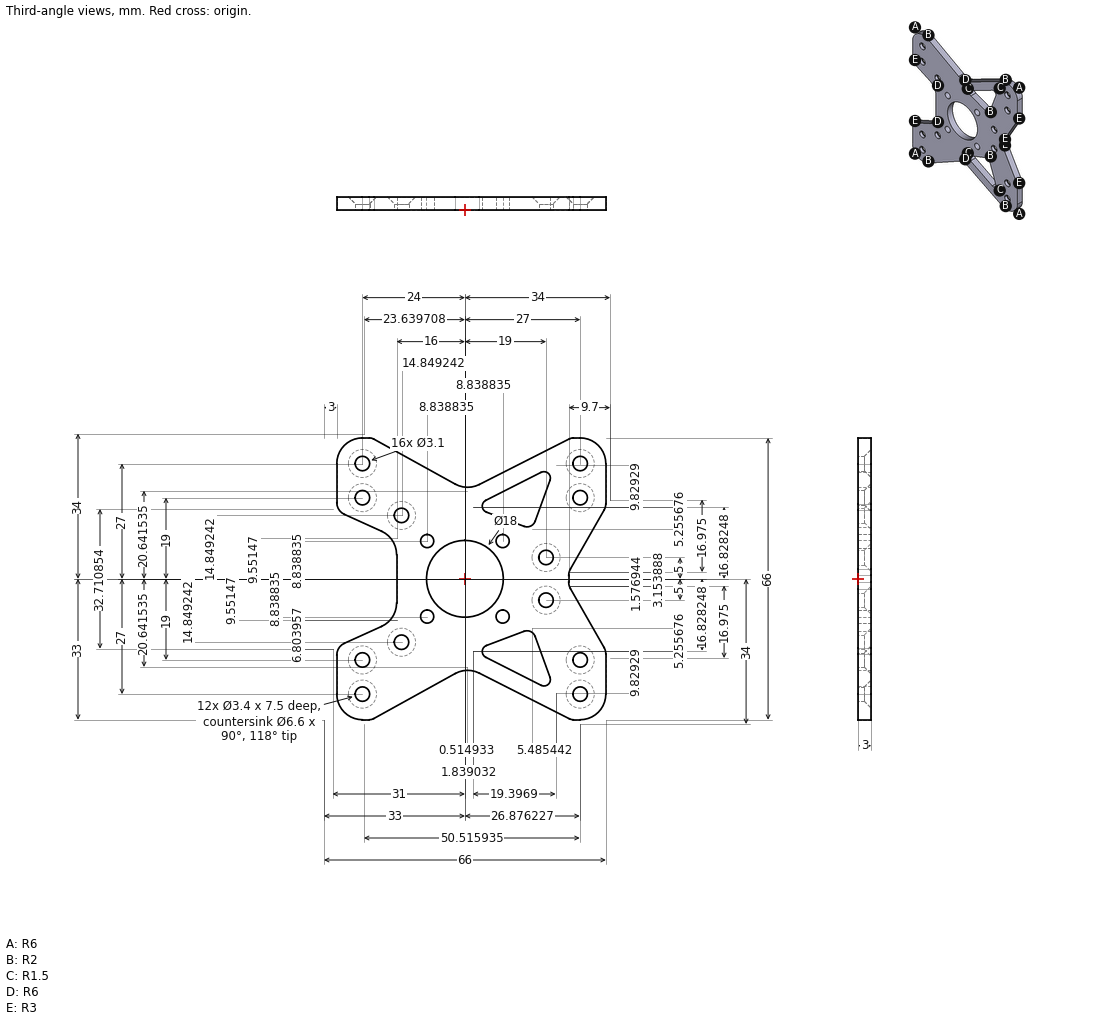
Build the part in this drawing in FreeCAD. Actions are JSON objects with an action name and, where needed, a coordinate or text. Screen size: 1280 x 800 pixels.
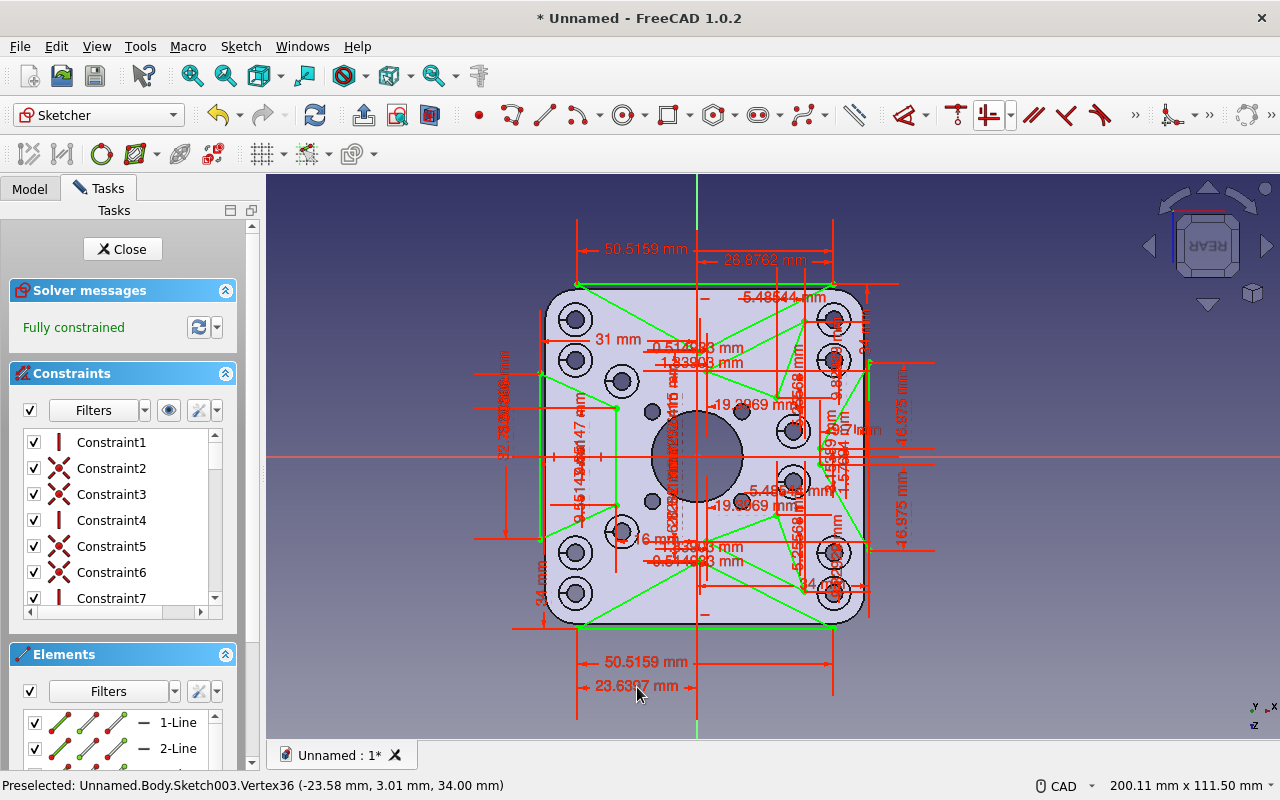
{"action": "left_click", "coordinate": [123, 249]}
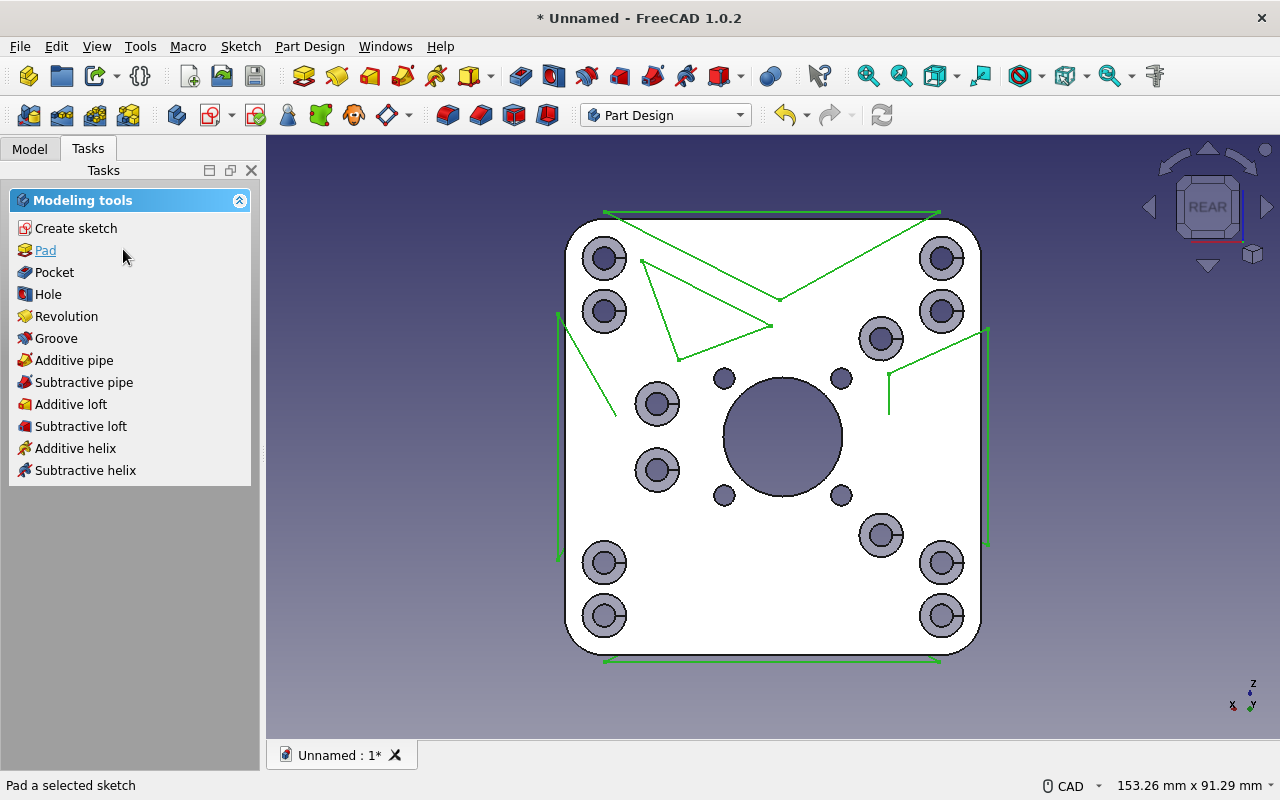
{"action": "left_click", "coordinate": [521, 76]}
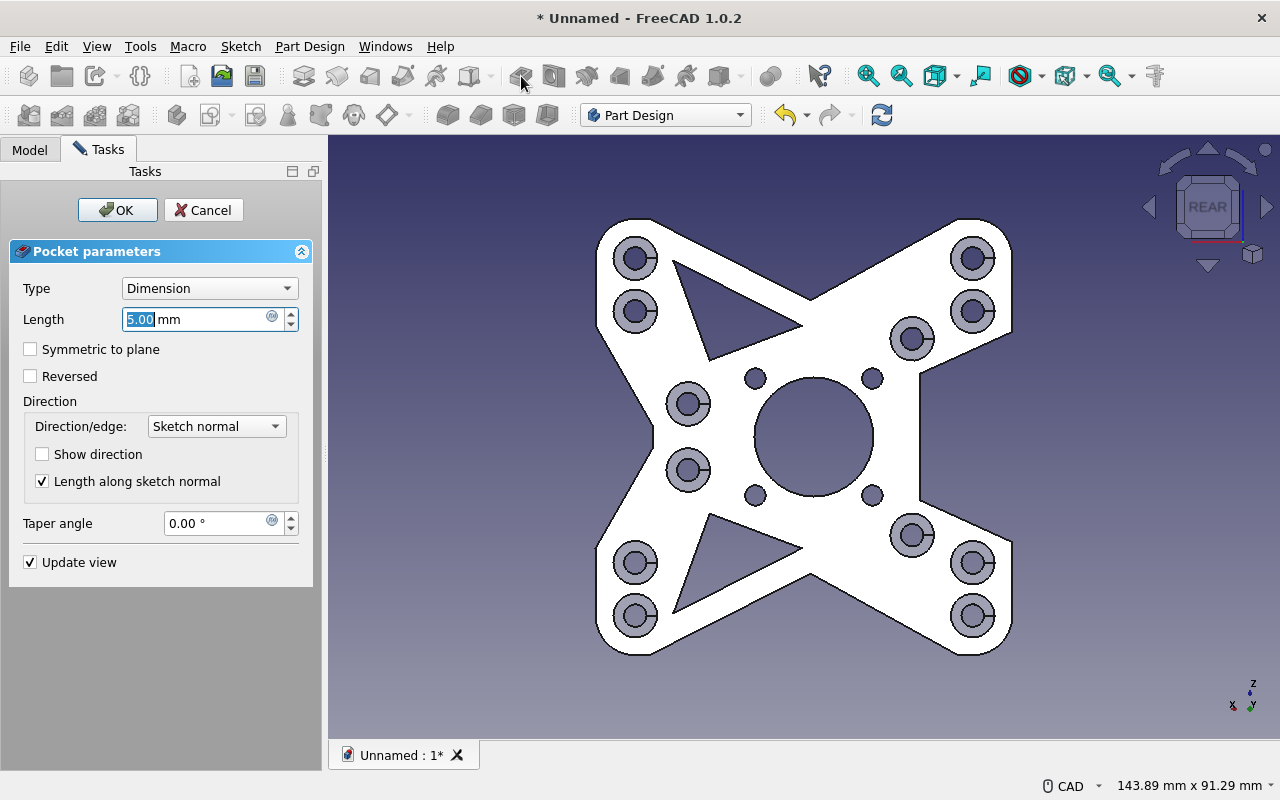
{"action": "left_click", "coordinate": [210, 288]}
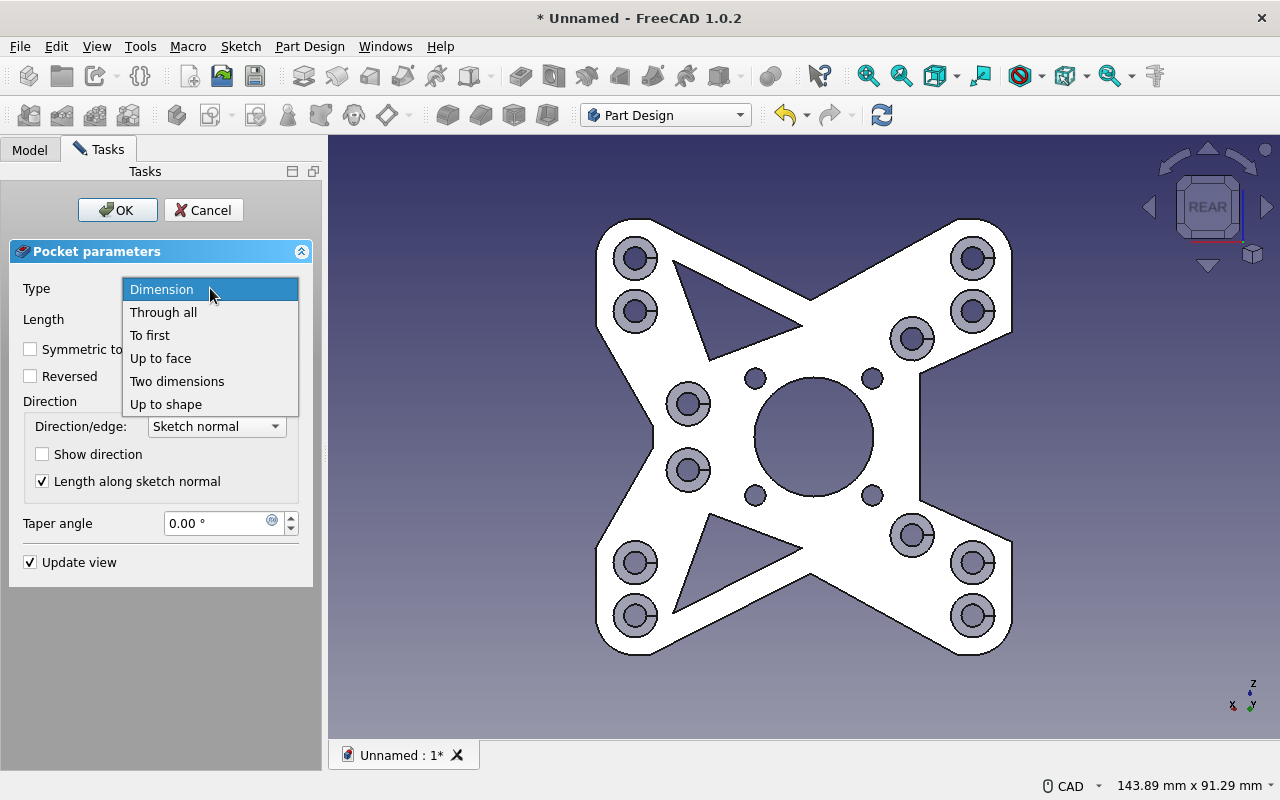
{"action": "left_click", "coordinate": [208, 312]}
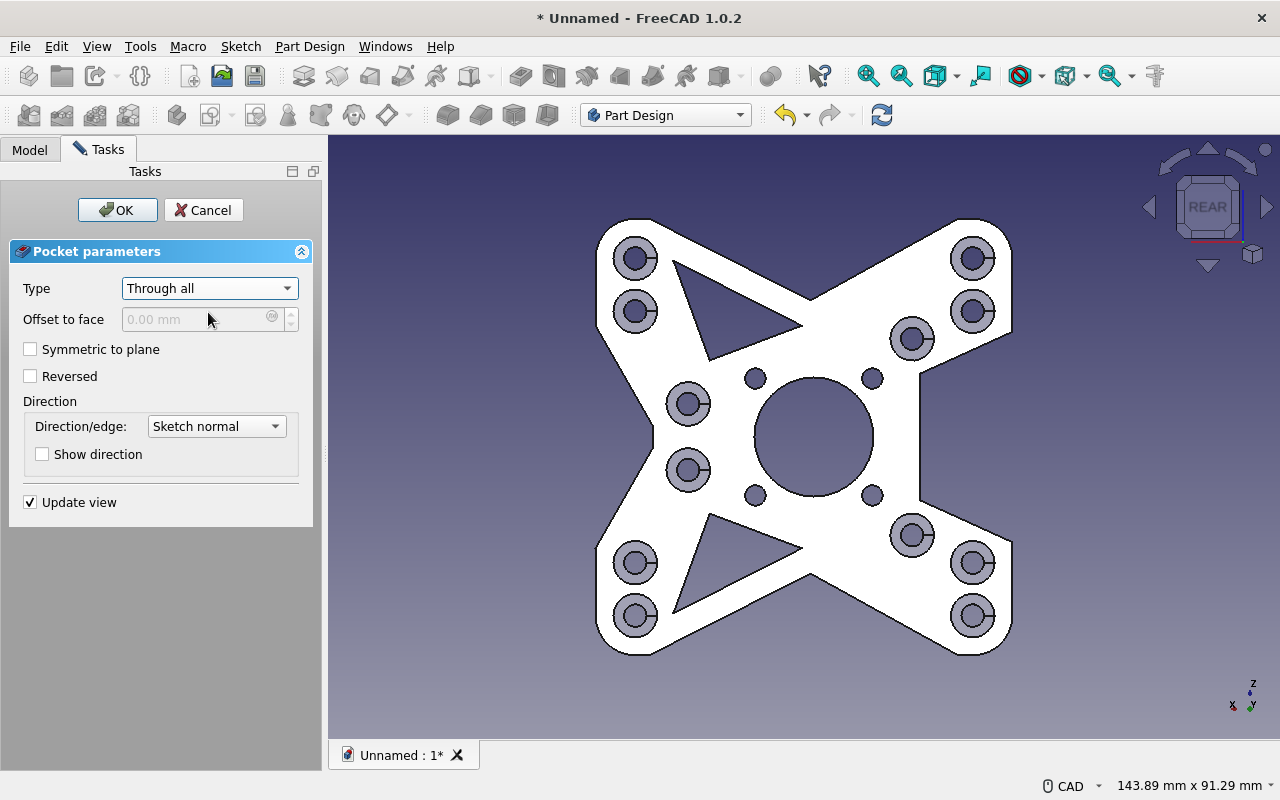
{"action": "left_click", "coordinate": [118, 210]}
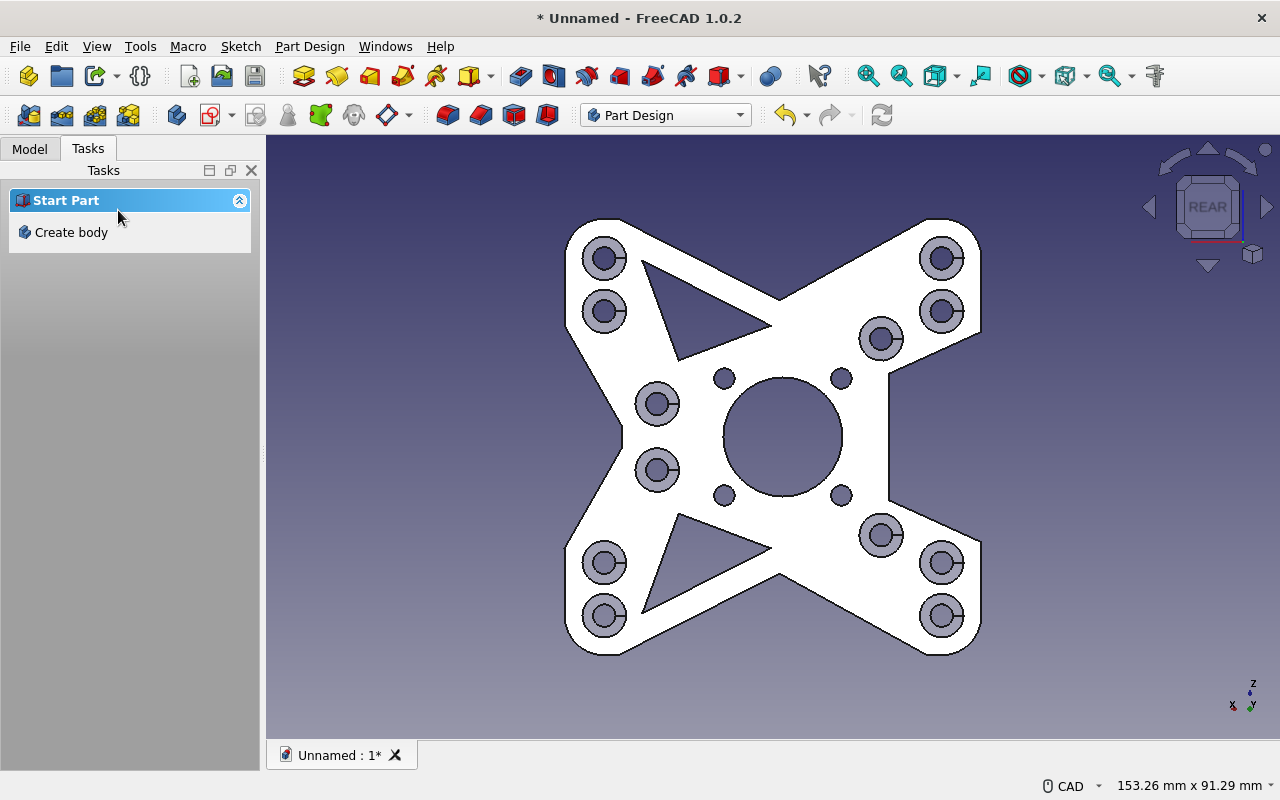
{"action": "scroll", "coordinate": [618, 218], "scroll_direction": "up", "scroll_amount": 4}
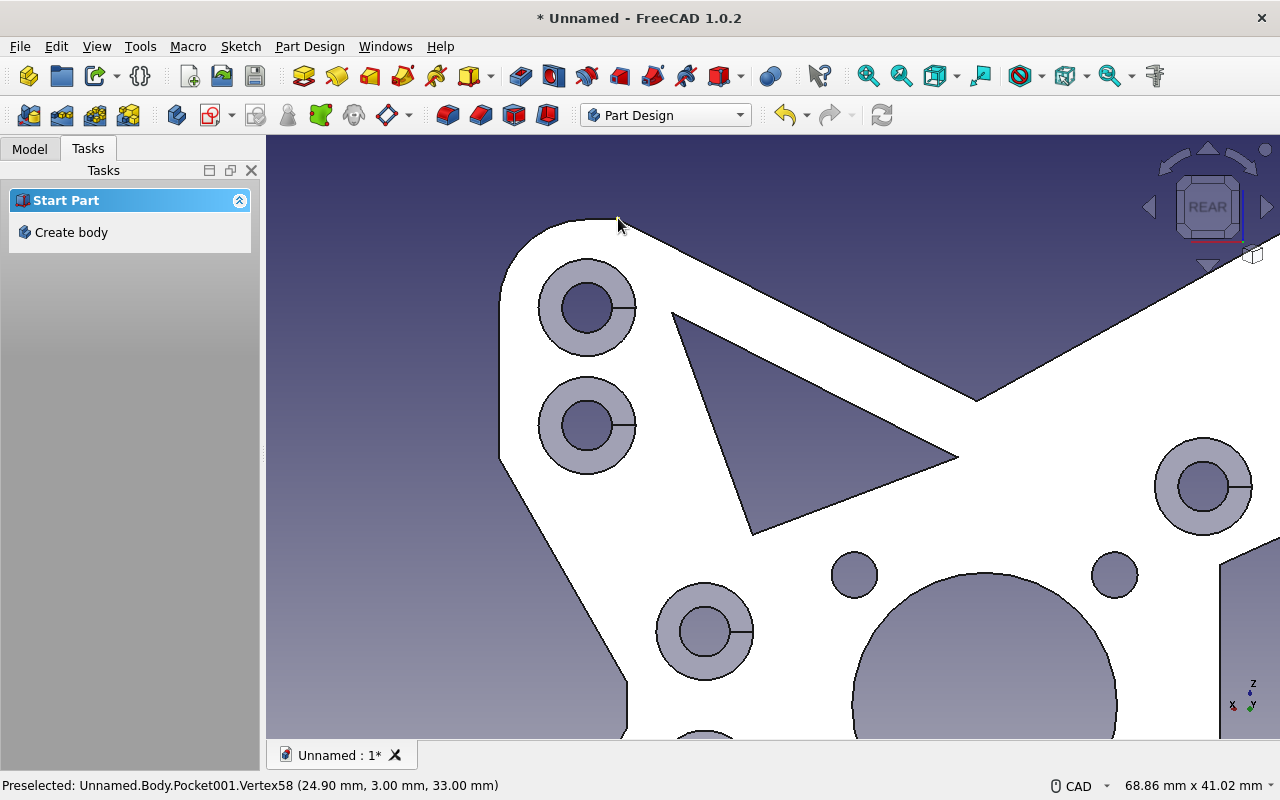
{"action": "left_click", "coordinate": [869, 76]}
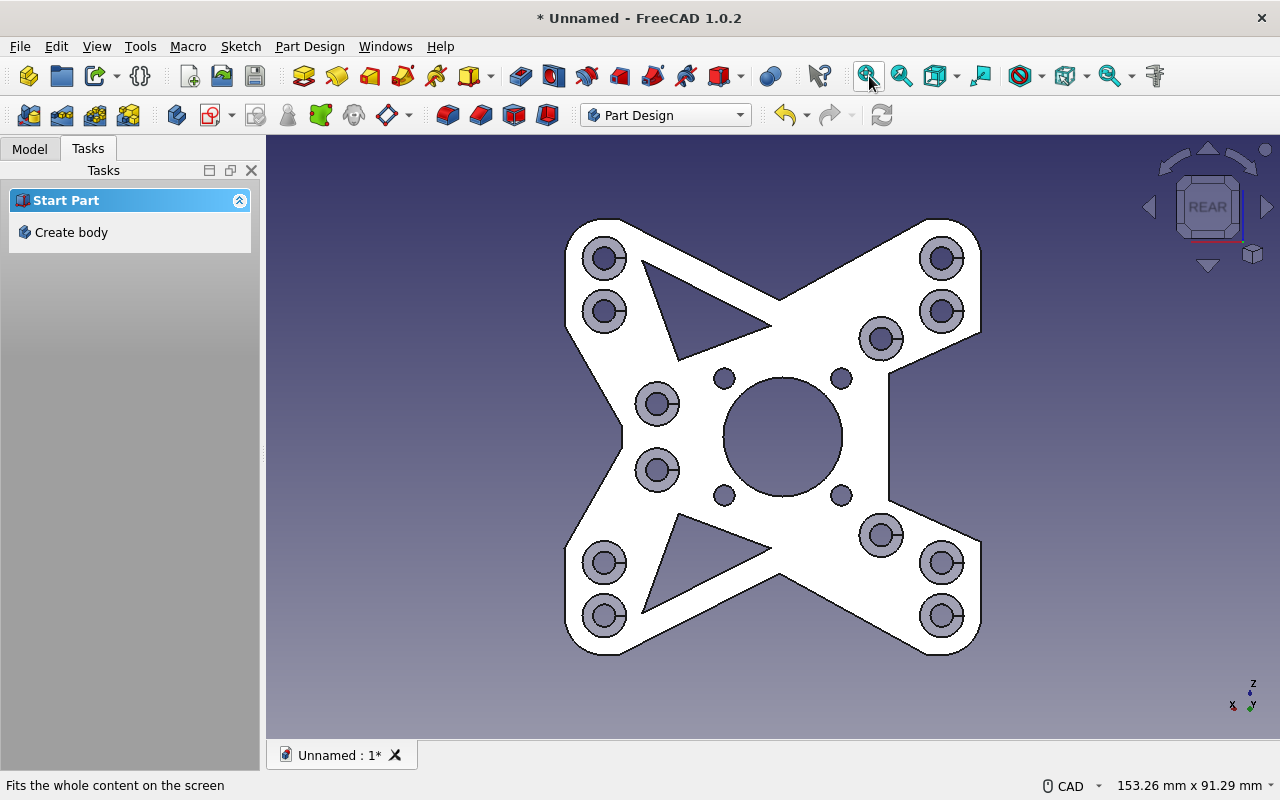
{"action": "key", "text": "0"}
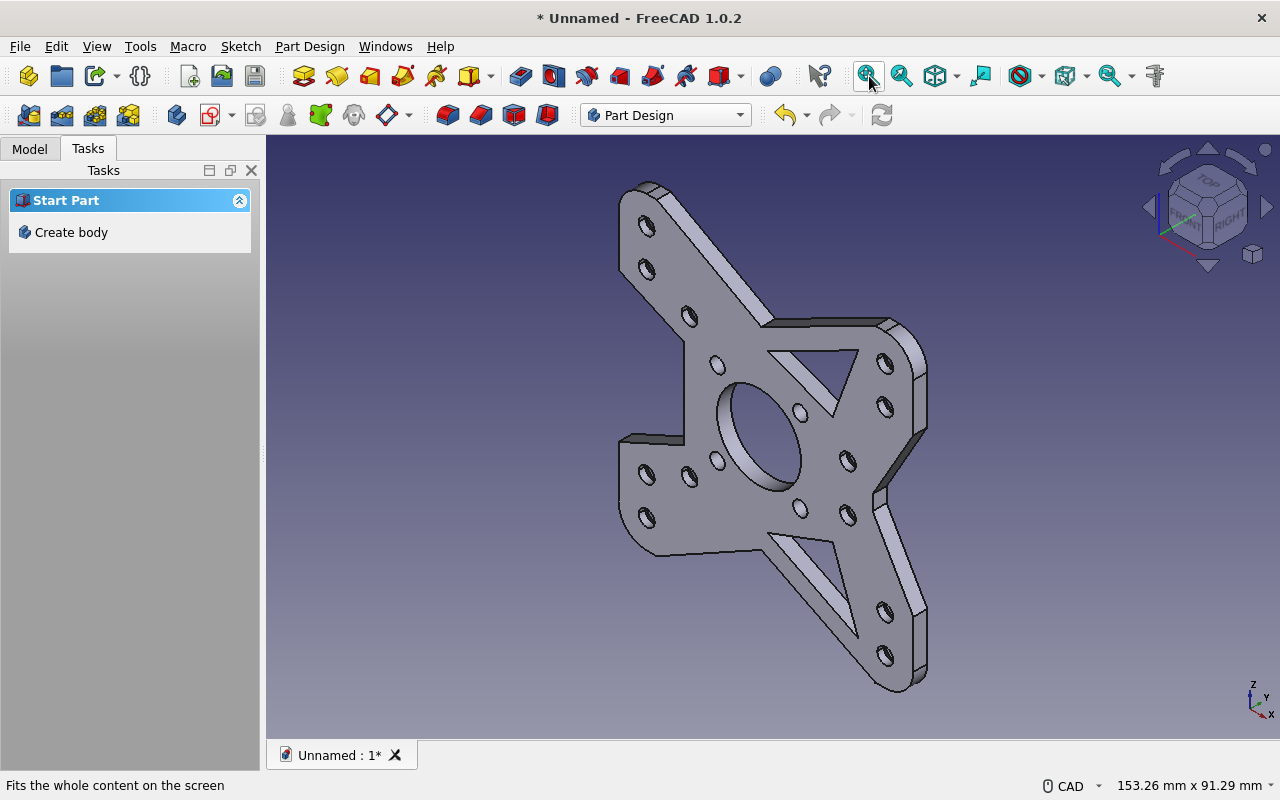
{"action": "scroll", "coordinate": [882, 321], "scroll_direction": "up", "scroll_amount": 4}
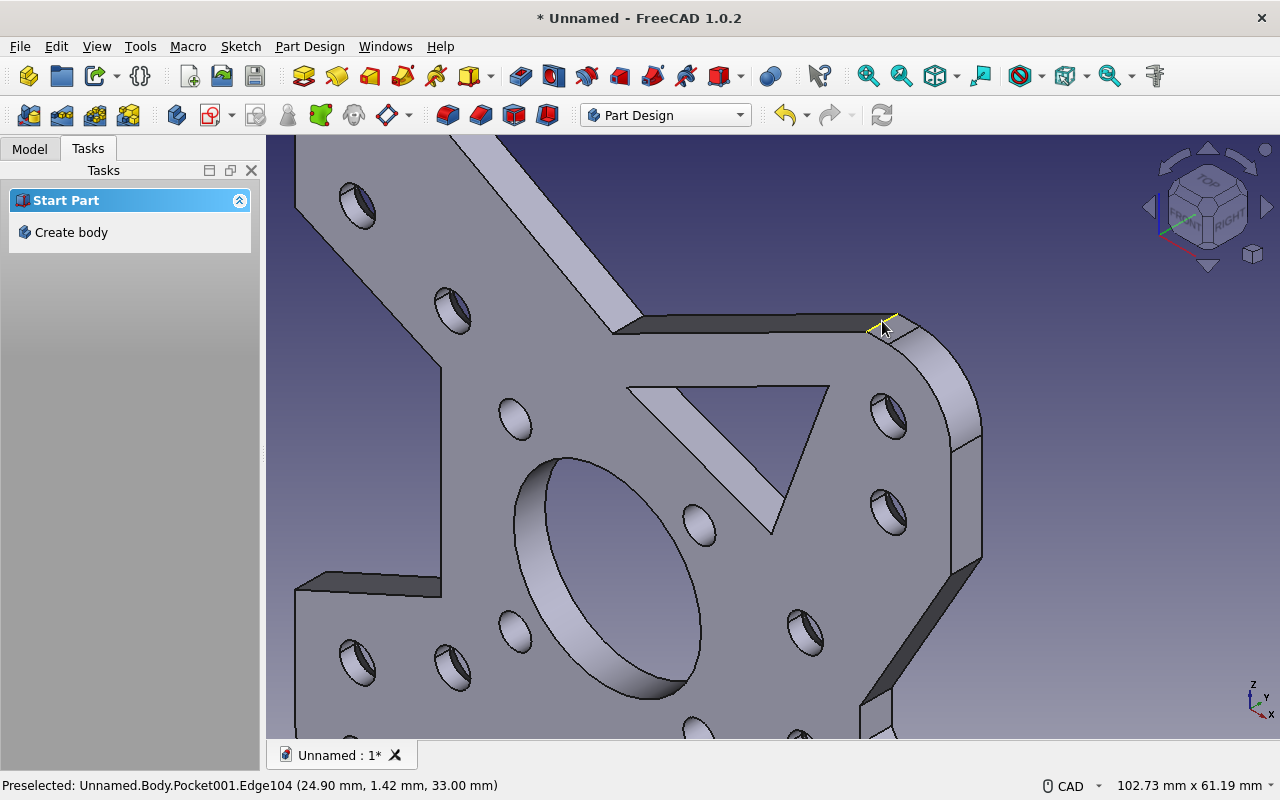
{"action": "left_click", "coordinate": [869, 76]}